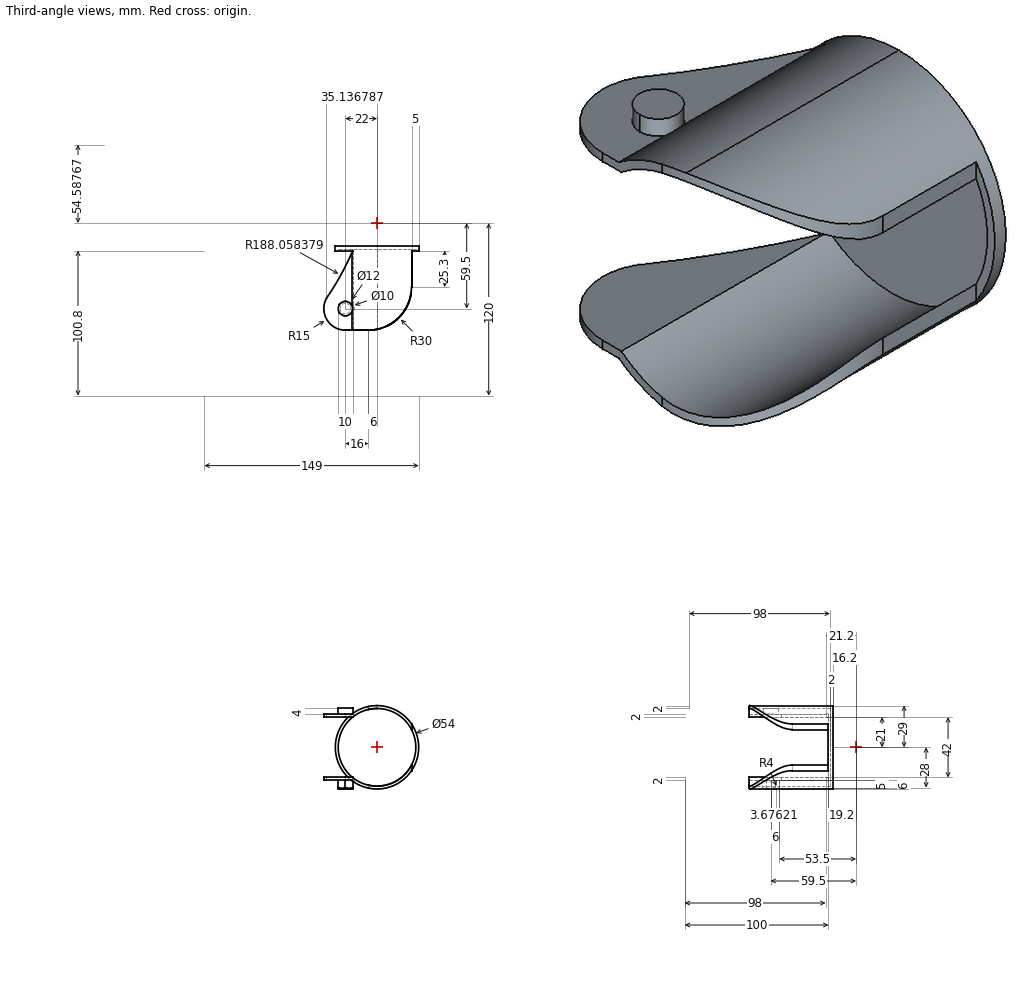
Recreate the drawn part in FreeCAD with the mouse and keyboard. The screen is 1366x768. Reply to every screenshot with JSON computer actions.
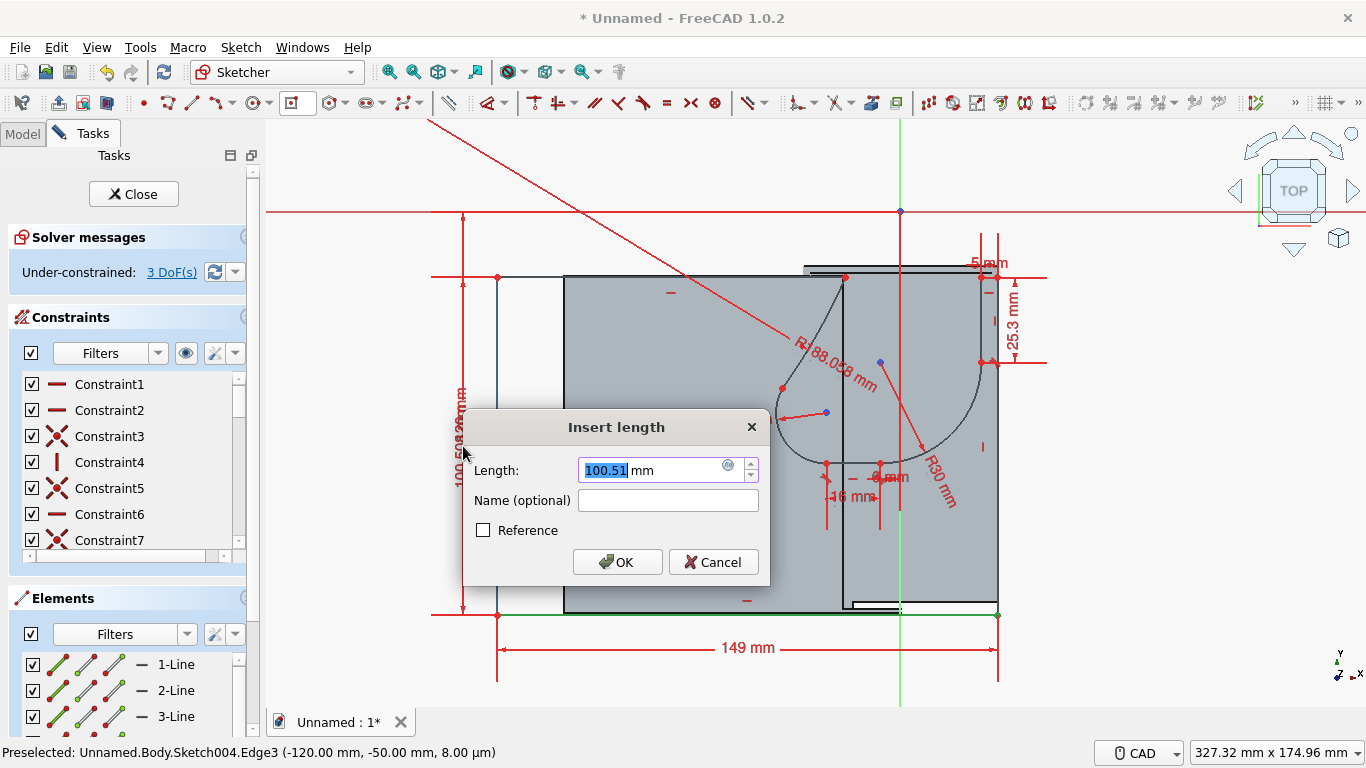
{"action": "type", "text": "100.8"}
{"action": "key", "text": "Return"}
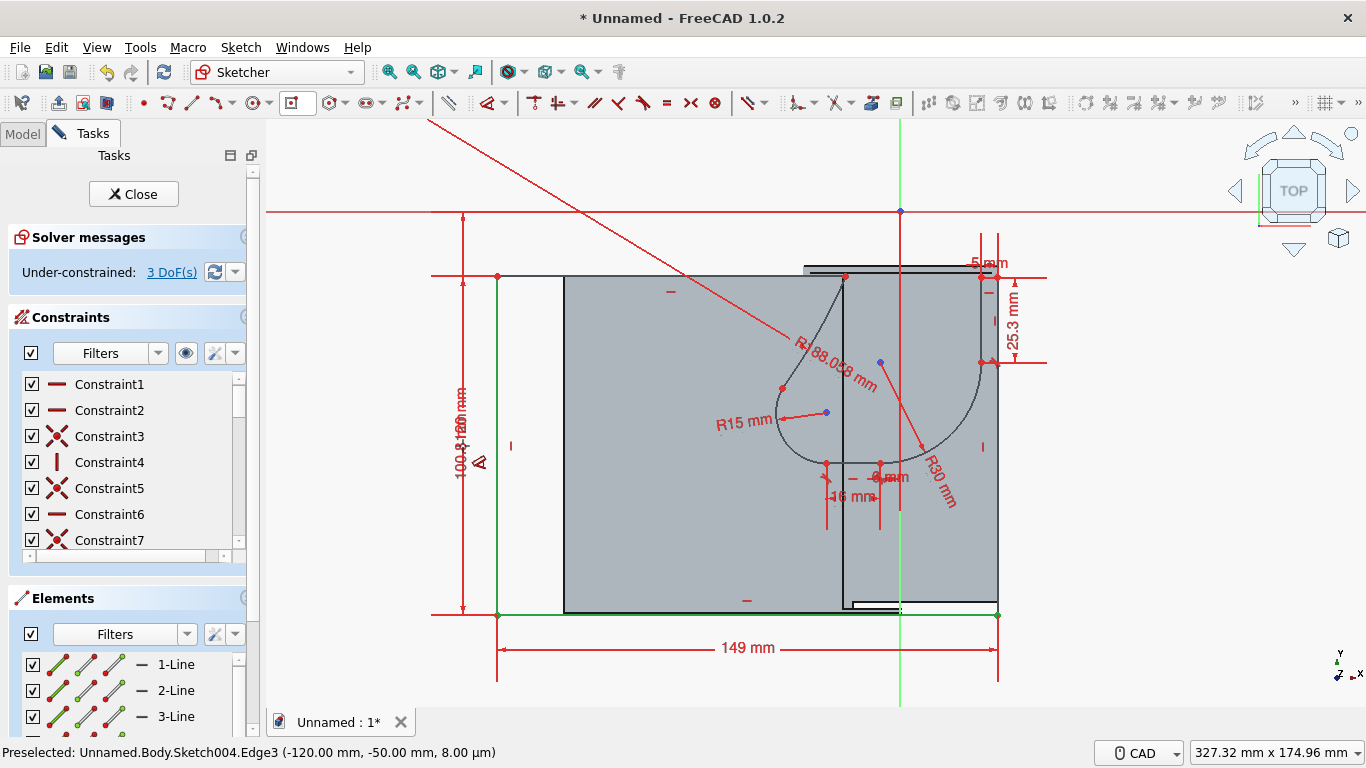
{"action": "left_click", "coordinate": [998, 514]}
{"action": "left_click", "coordinate": [1032, 446]}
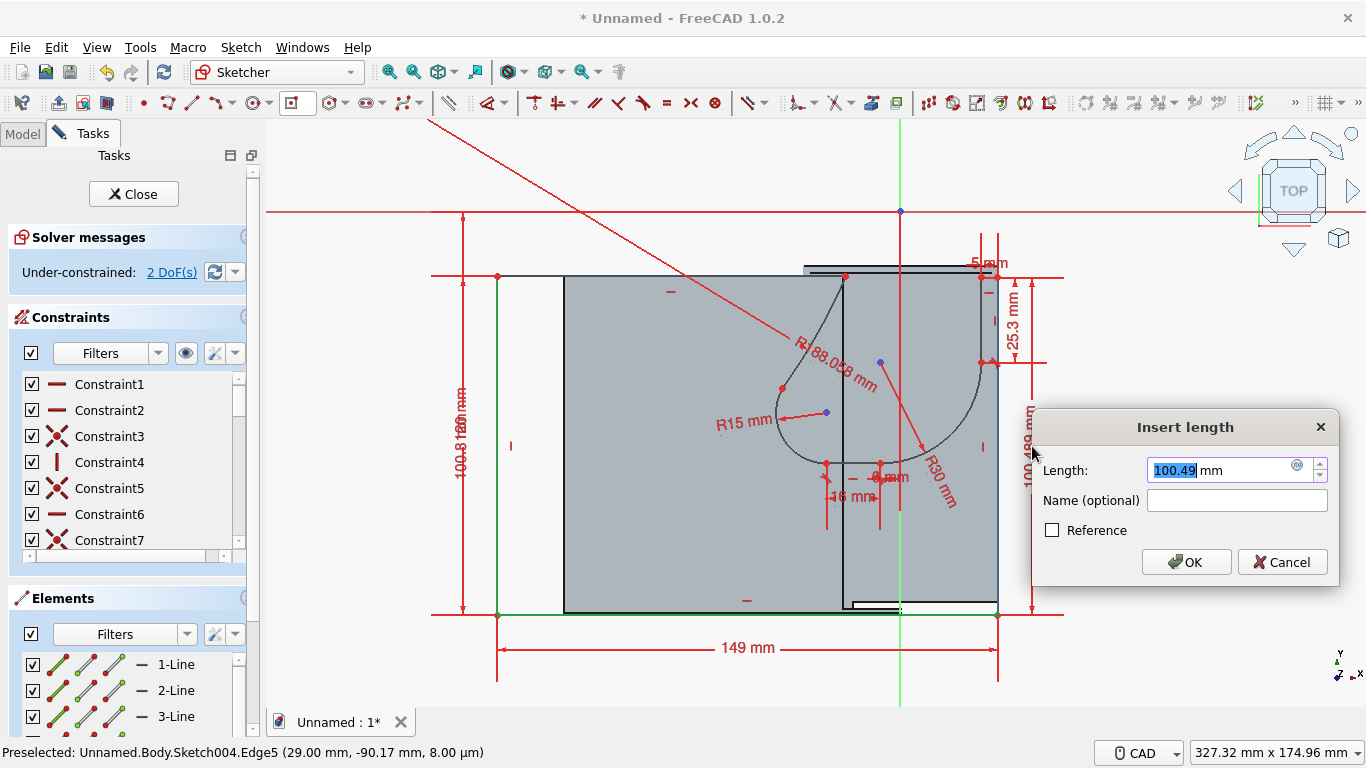
{"action": "type", "text": "100.8"}
{"action": "key", "text": "Return"}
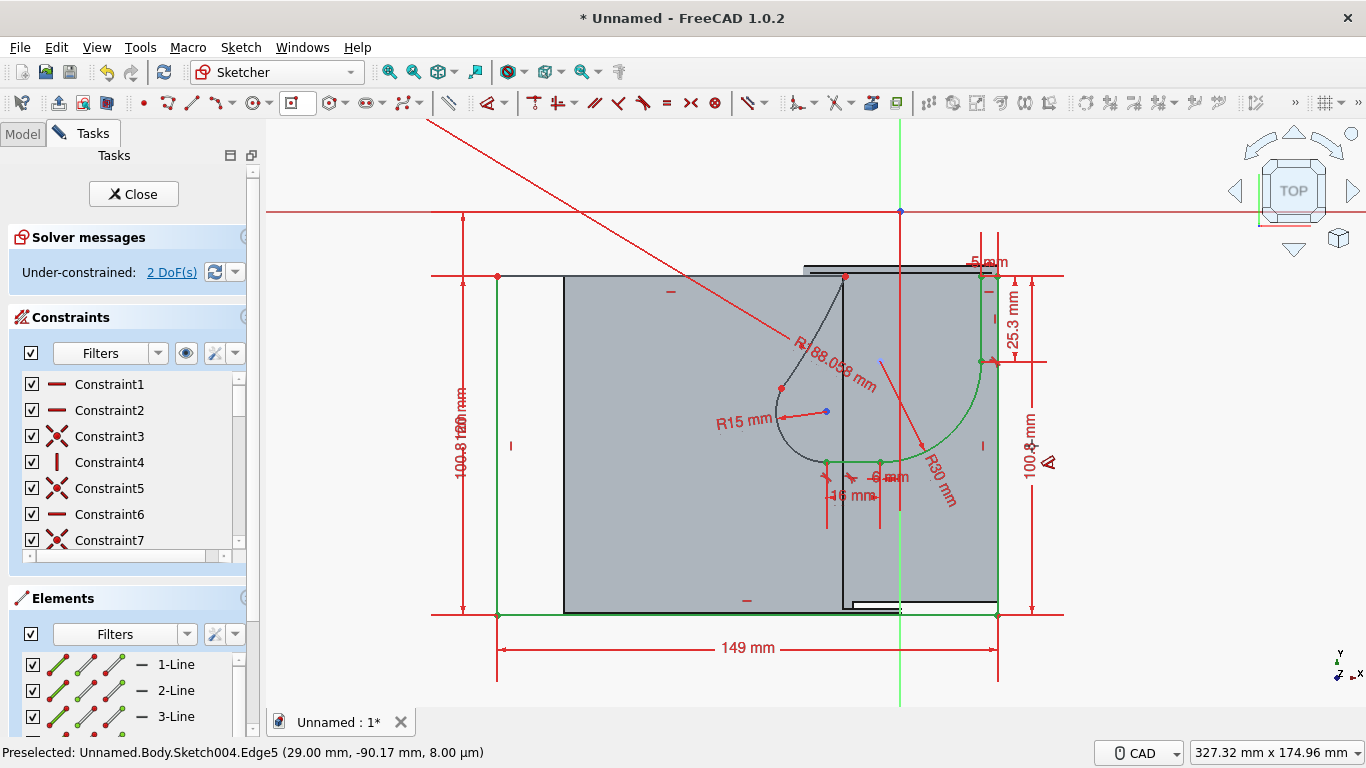
{"action": "scroll", "coordinate": [982, 604], "scroll_direction": "down", "scroll_amount": 2}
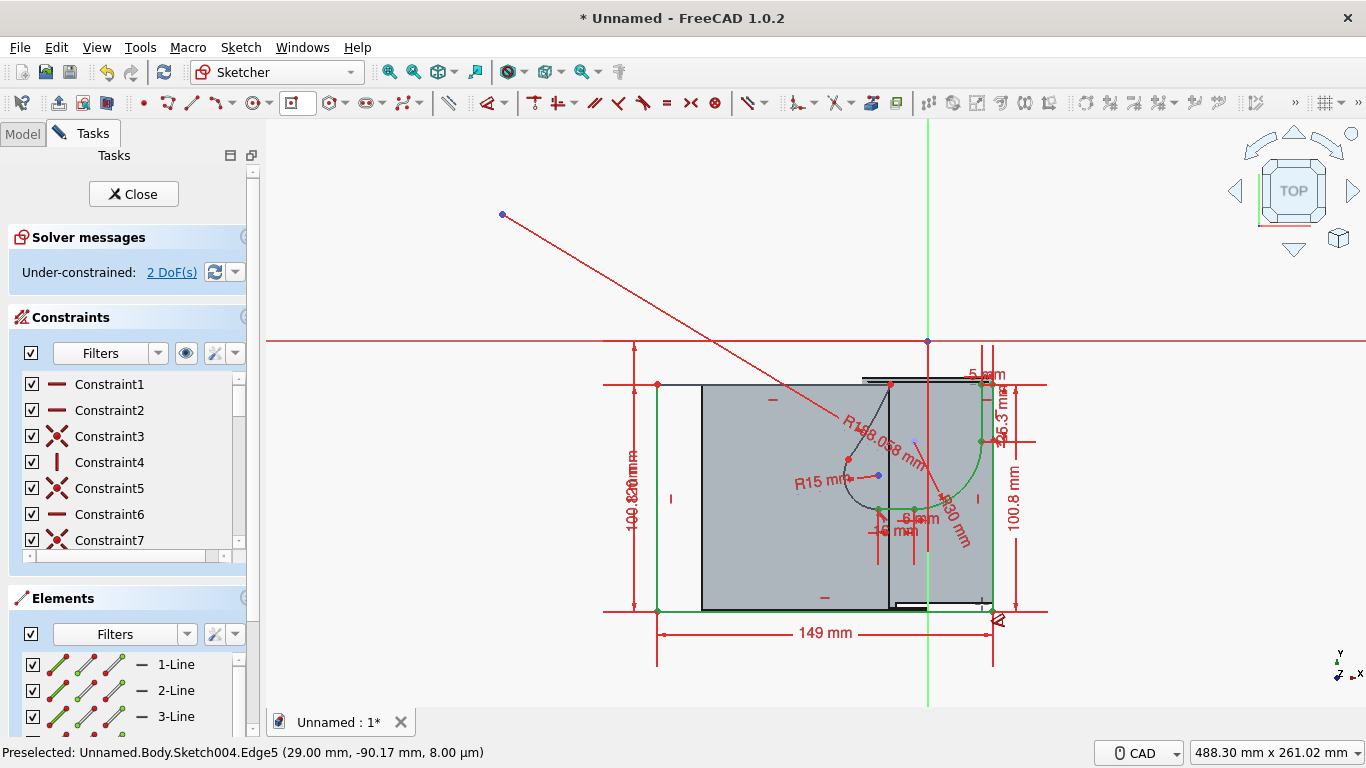
{"action": "left_click", "coordinate": [503, 214]}
{"action": "left_click", "coordinate": [469, 278]}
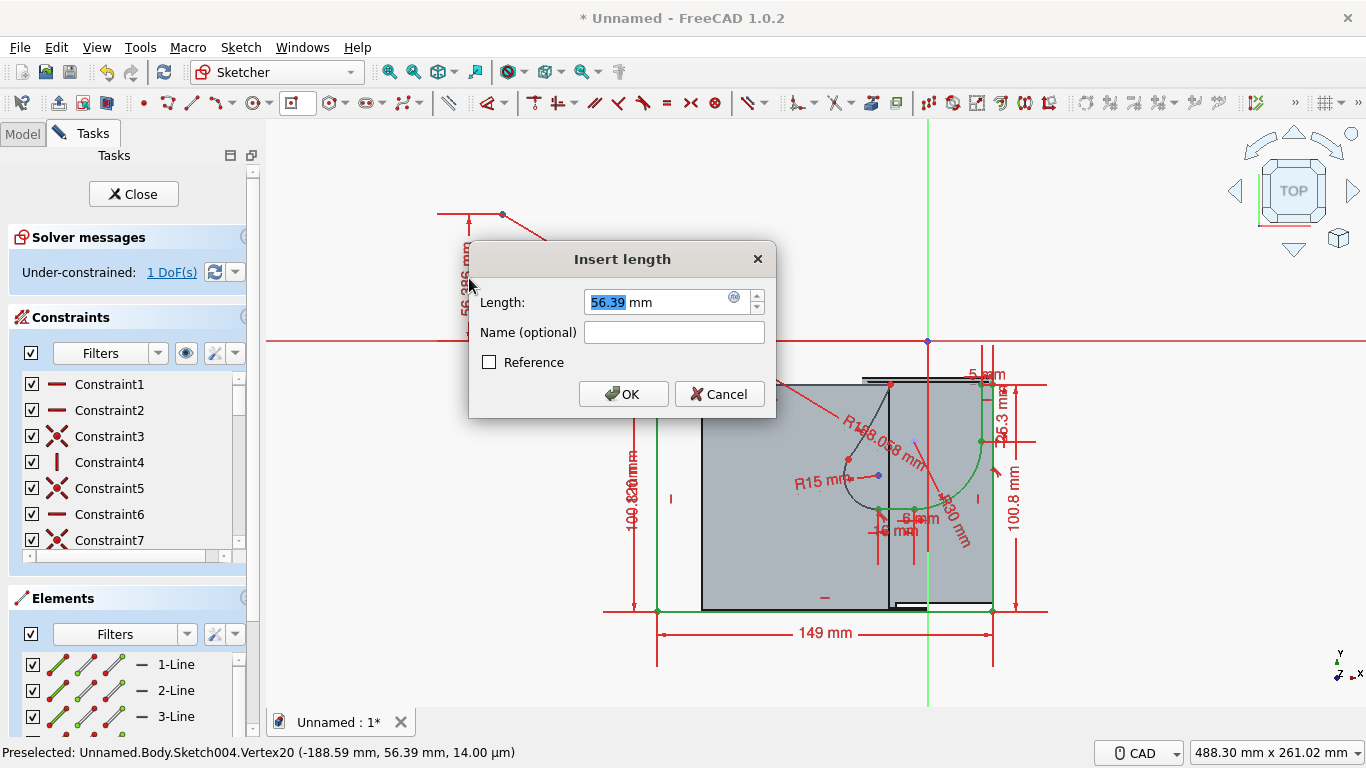
{"action": "type", "text": "54.58767"}
{"action": "key", "text": "Return"}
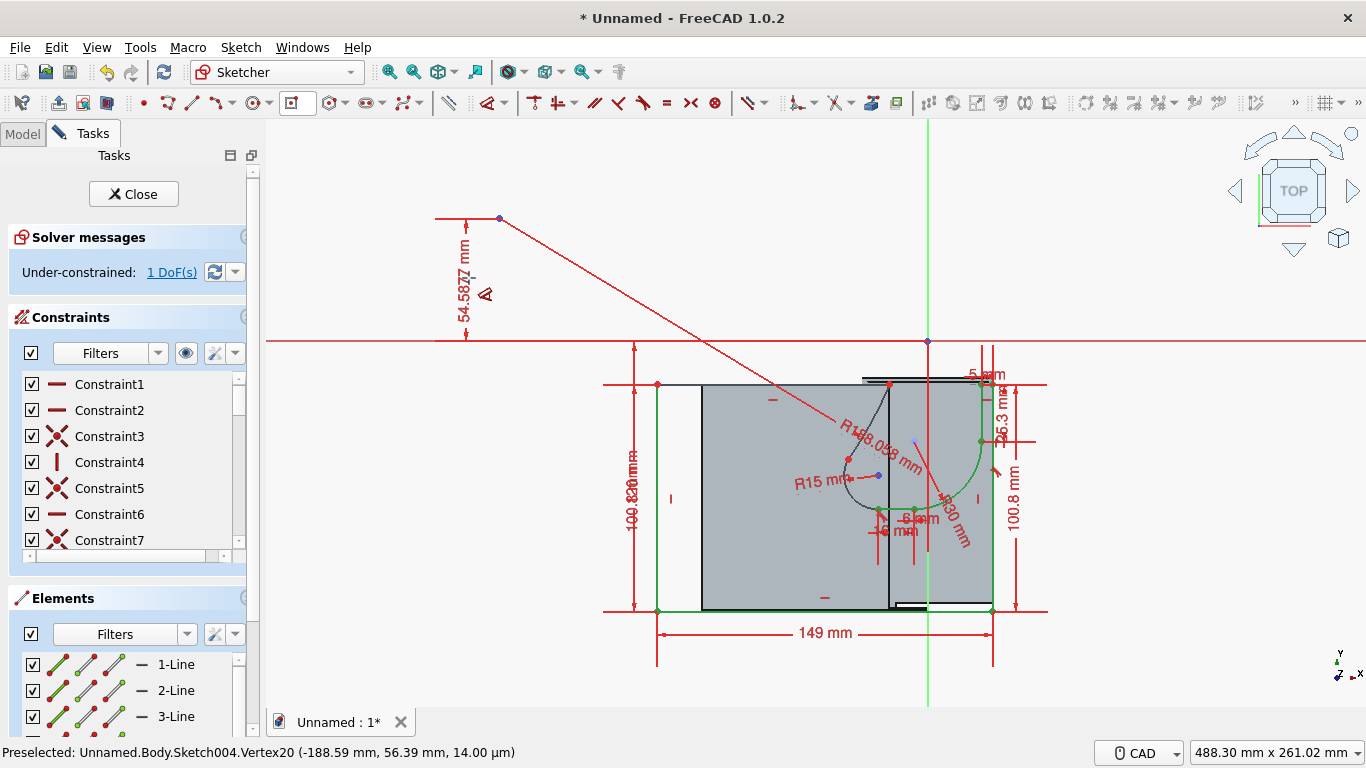
{"action": "left_click", "coordinate": [848, 460]}
{"action": "left_click", "coordinate": [888, 307]}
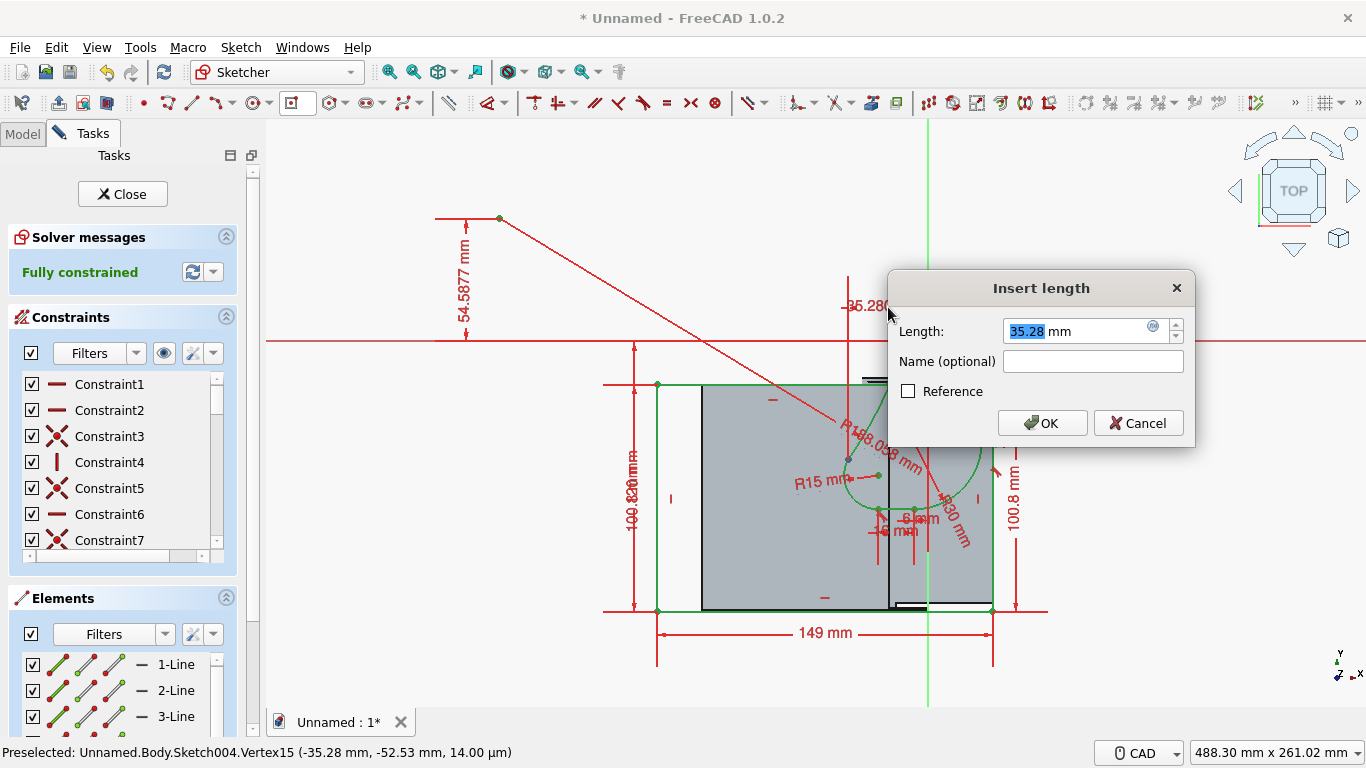
{"action": "type", "text": "35.136787"}
{"action": "key", "text": "Return"}
{"action": "key", "text": "Escape"}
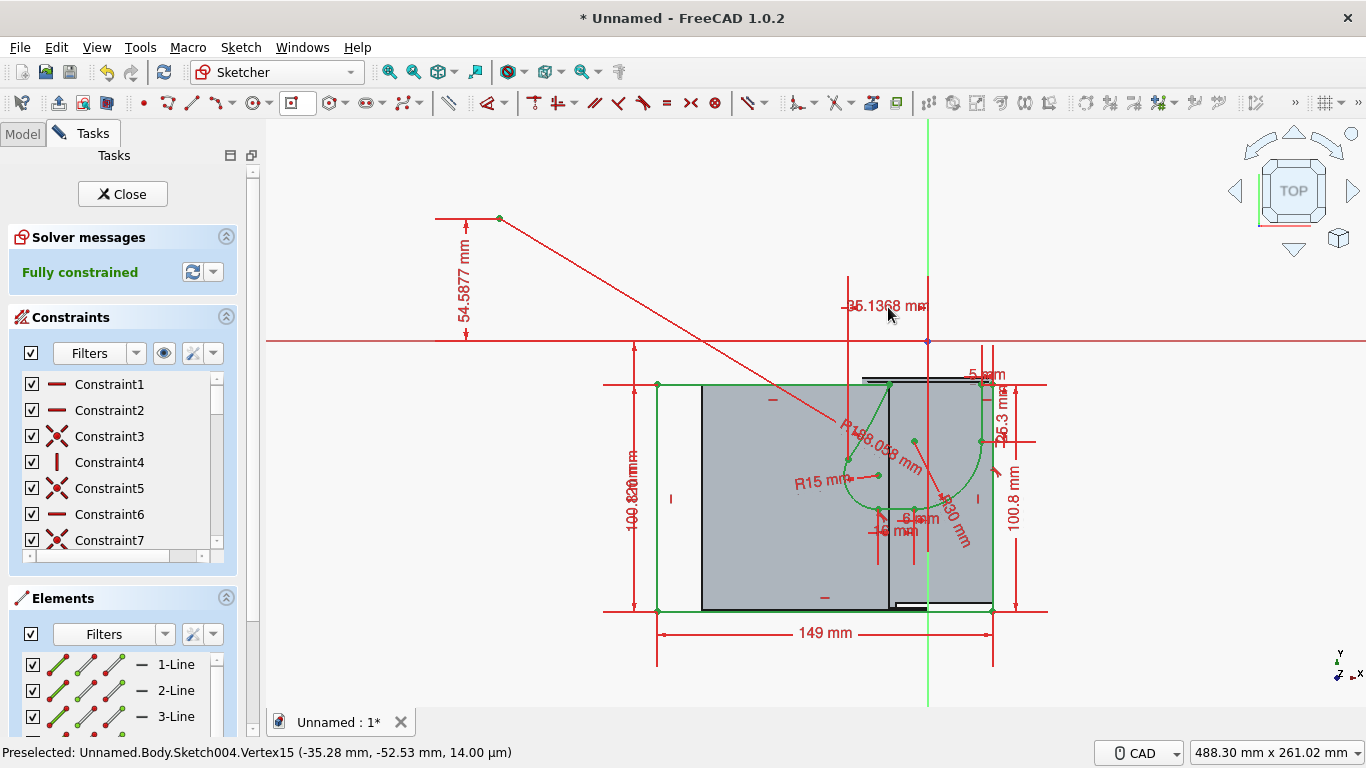
{"action": "left_click", "coordinate": [123, 194]}